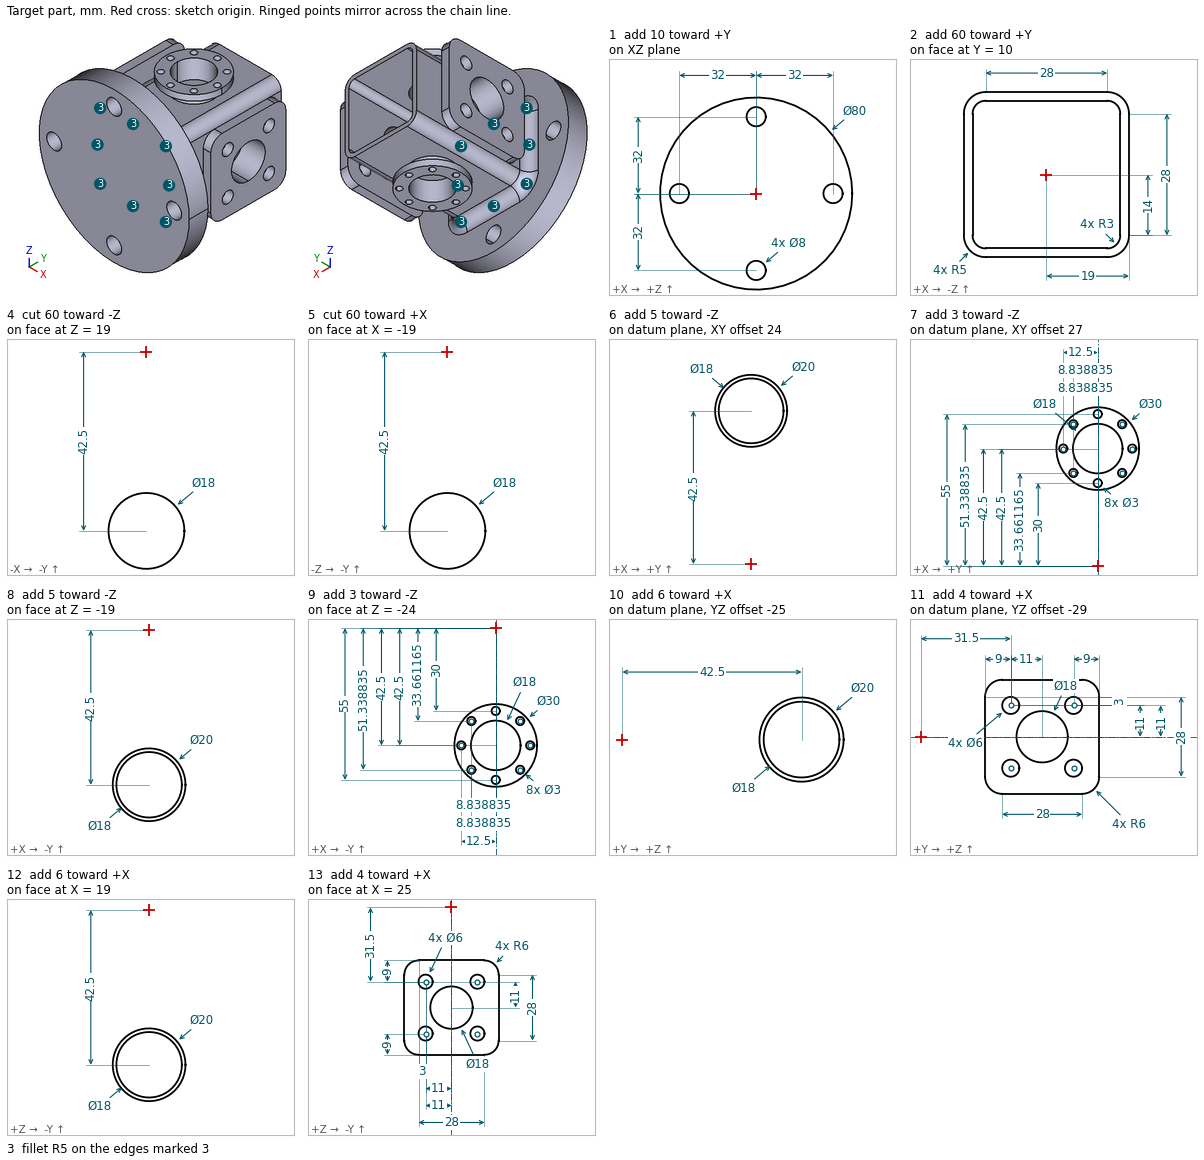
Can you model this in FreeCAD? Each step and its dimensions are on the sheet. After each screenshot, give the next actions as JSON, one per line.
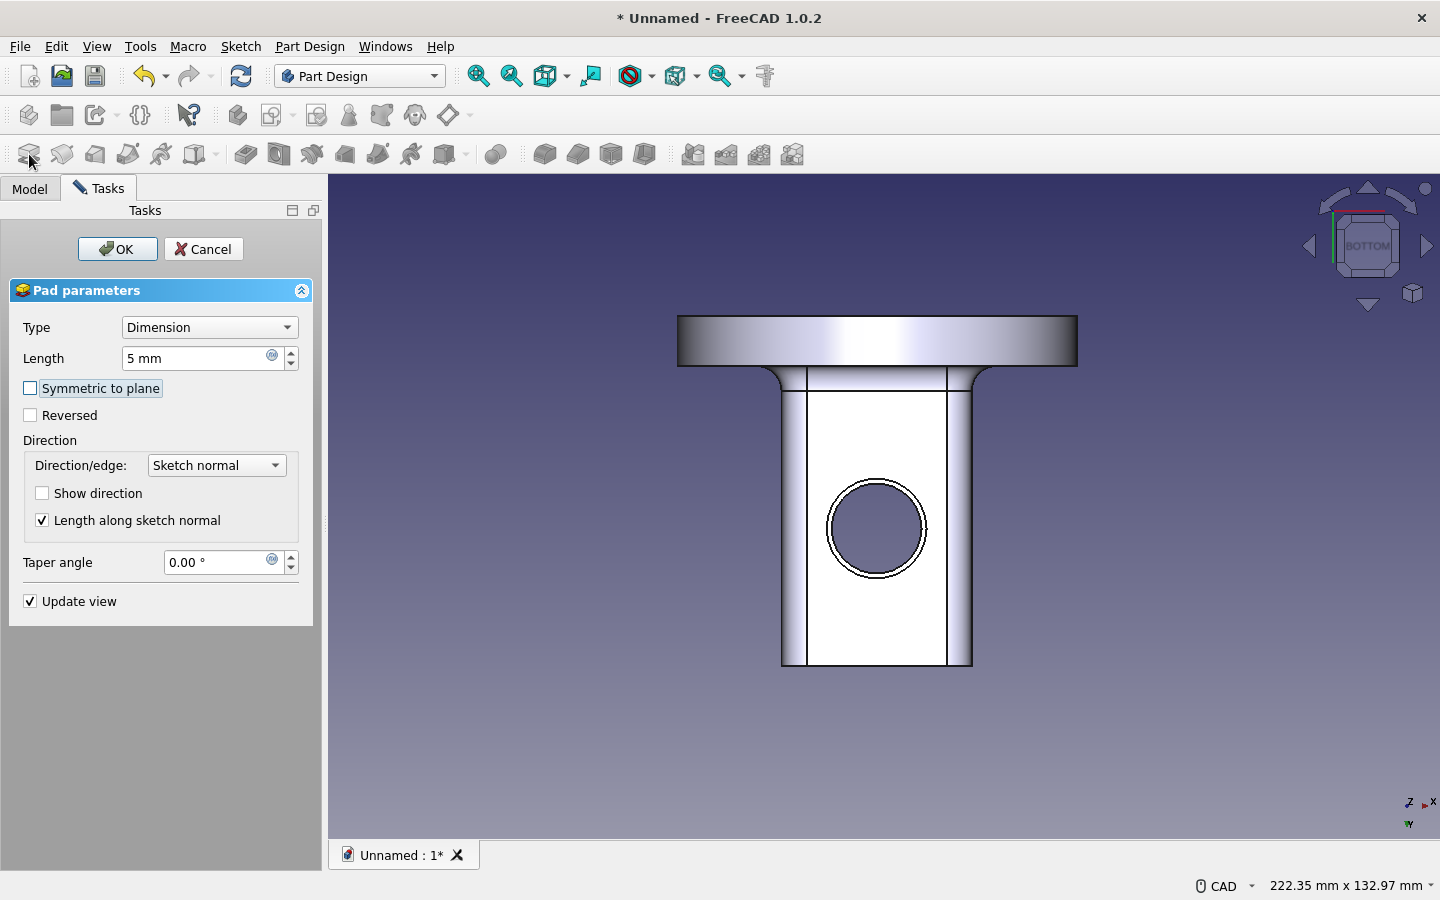
{"action": "left_click", "coordinate": [118, 249]}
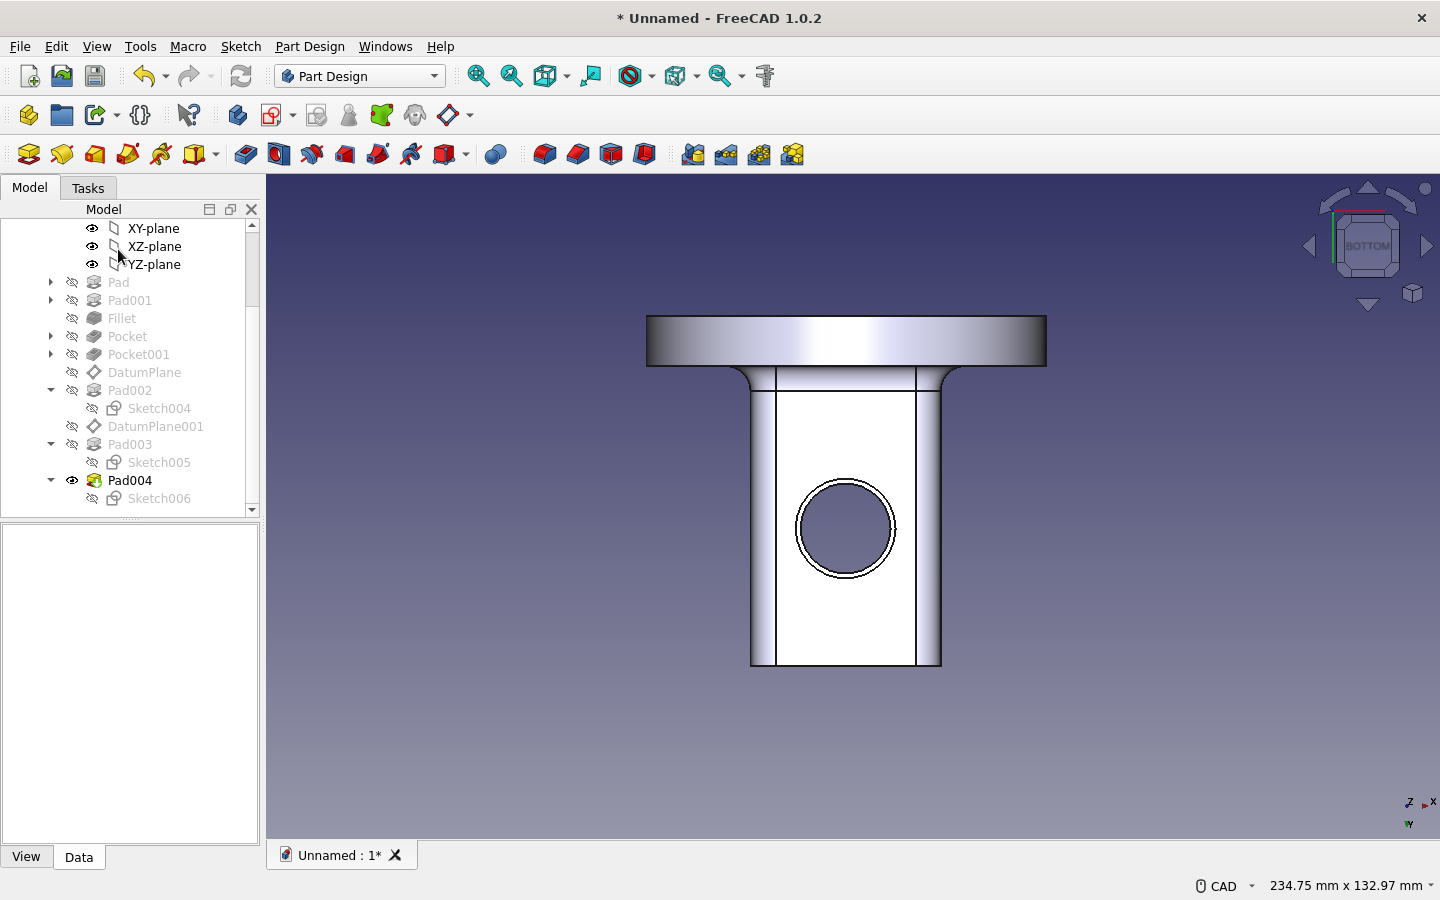
{"action": "scroll", "coordinate": [831, 570], "scroll_direction": "up", "scroll_amount": 15}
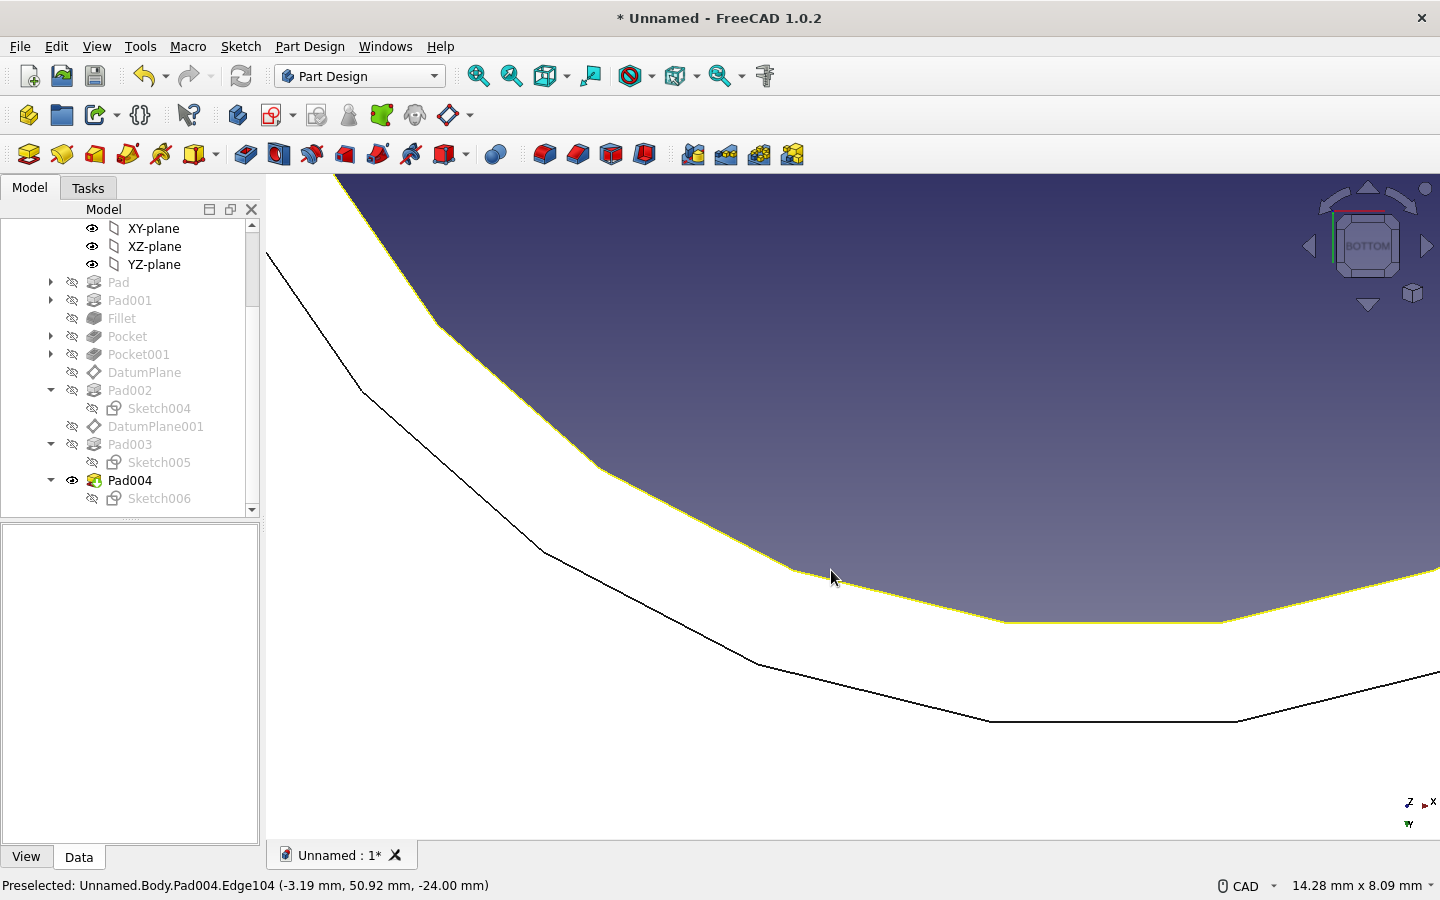
{"action": "scroll", "coordinate": [827, 585], "scroll_direction": "up", "scroll_amount": 7}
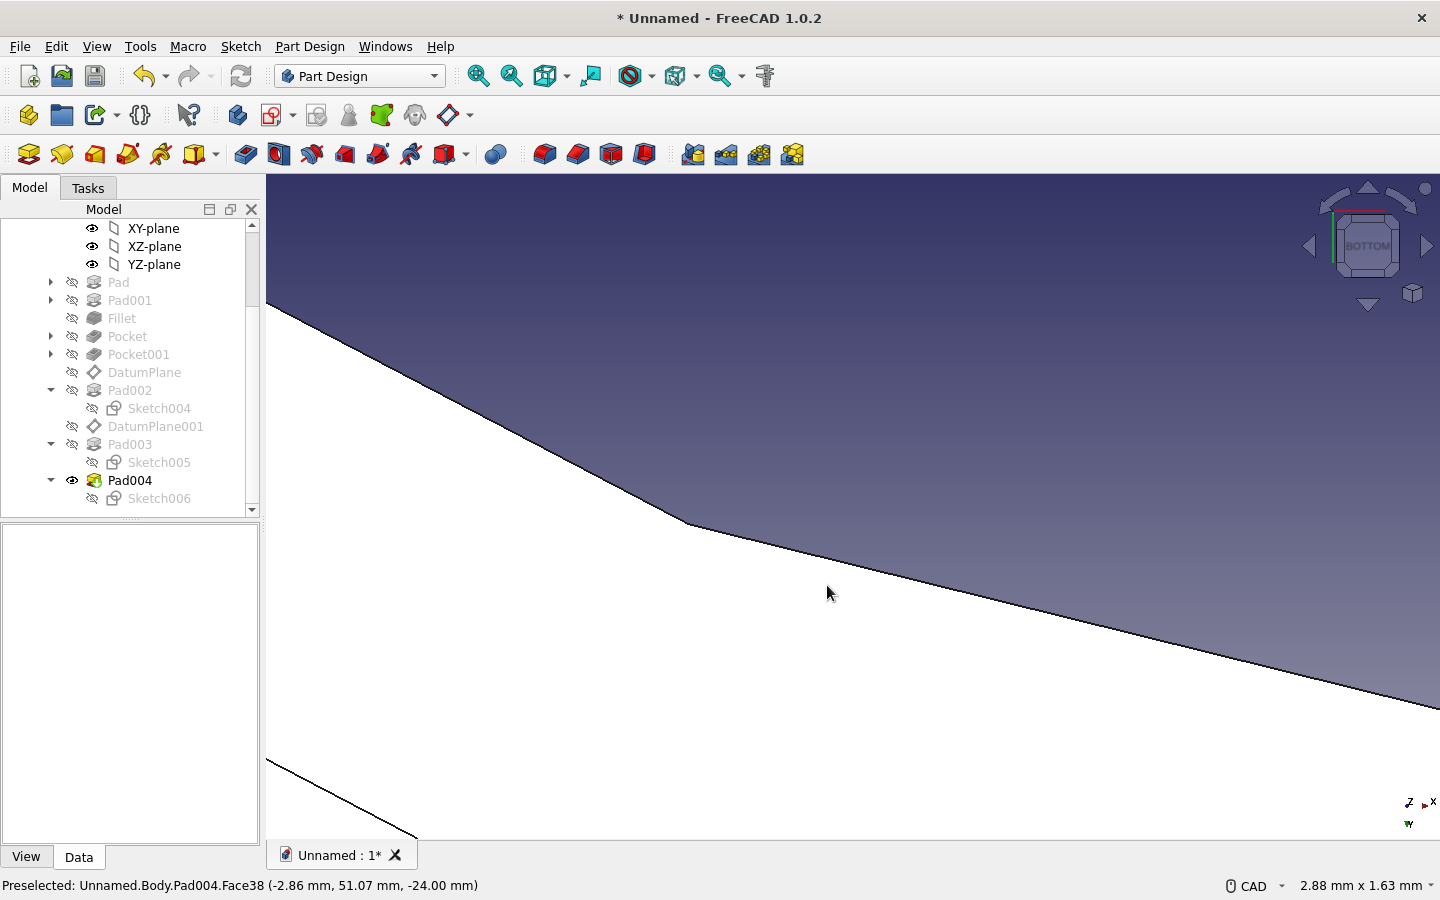
{"action": "left_click", "coordinate": [825, 587]}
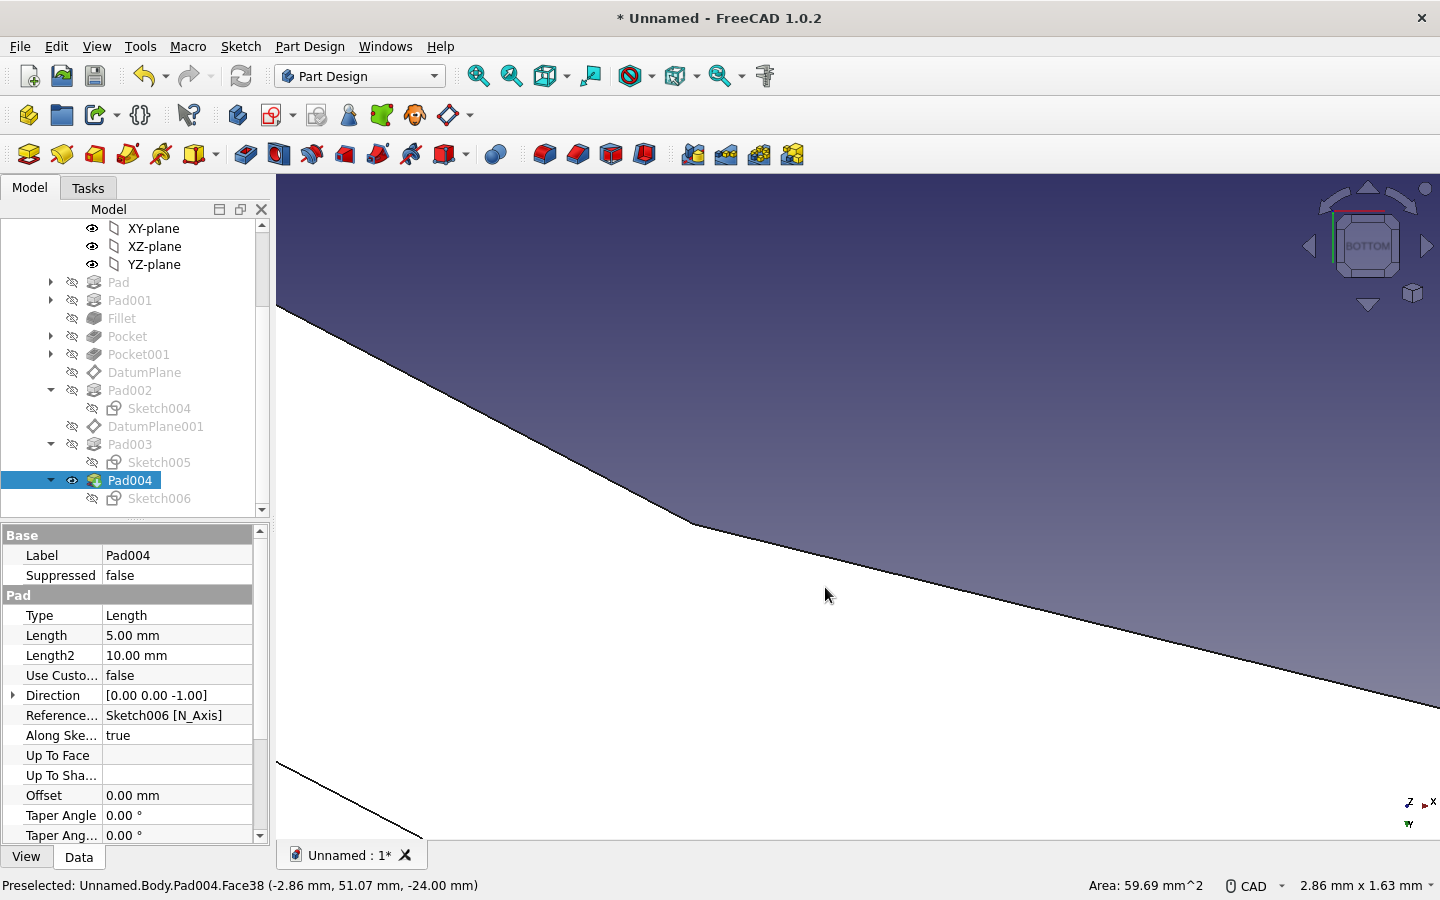
{"action": "left_click", "coordinate": [270, 116]}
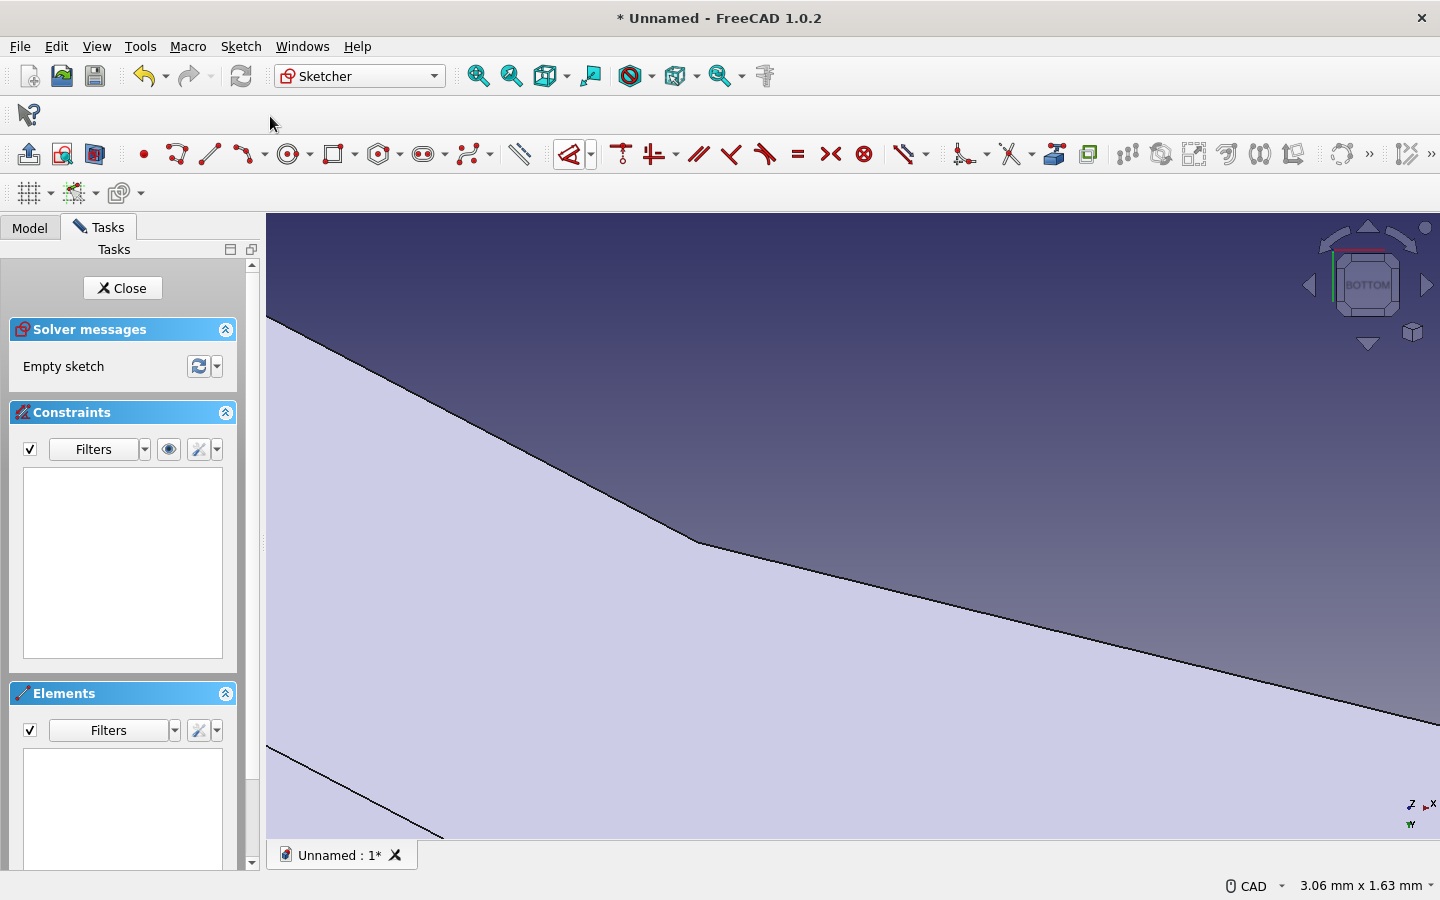
{"action": "scroll", "coordinate": [784, 526], "scroll_direction": "down", "scroll_amount": 15}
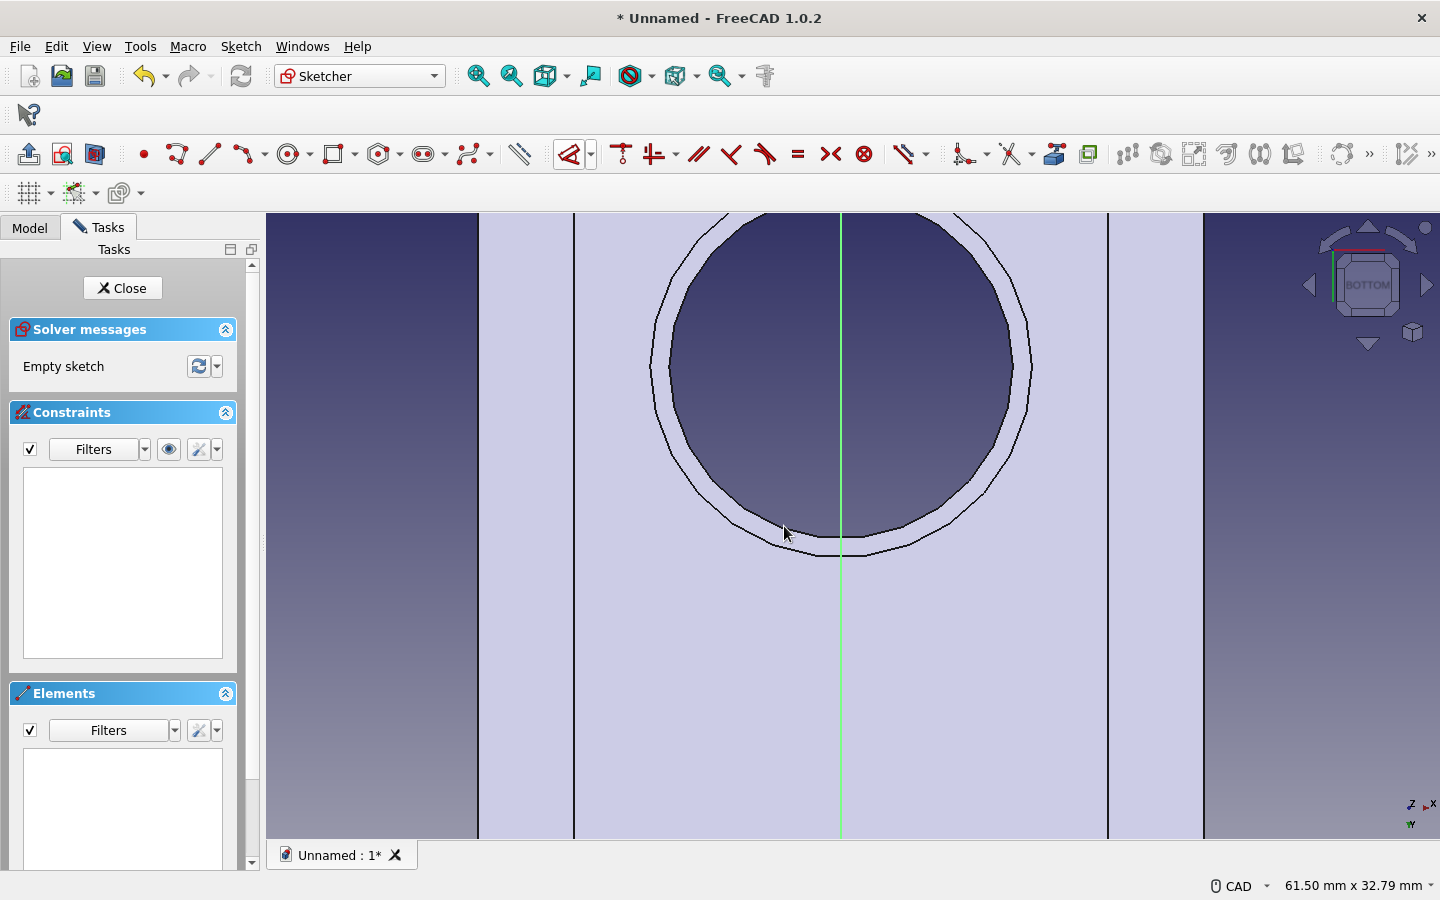
{"action": "scroll", "coordinate": [752, 772], "scroll_direction": "down", "scroll_amount": 5}